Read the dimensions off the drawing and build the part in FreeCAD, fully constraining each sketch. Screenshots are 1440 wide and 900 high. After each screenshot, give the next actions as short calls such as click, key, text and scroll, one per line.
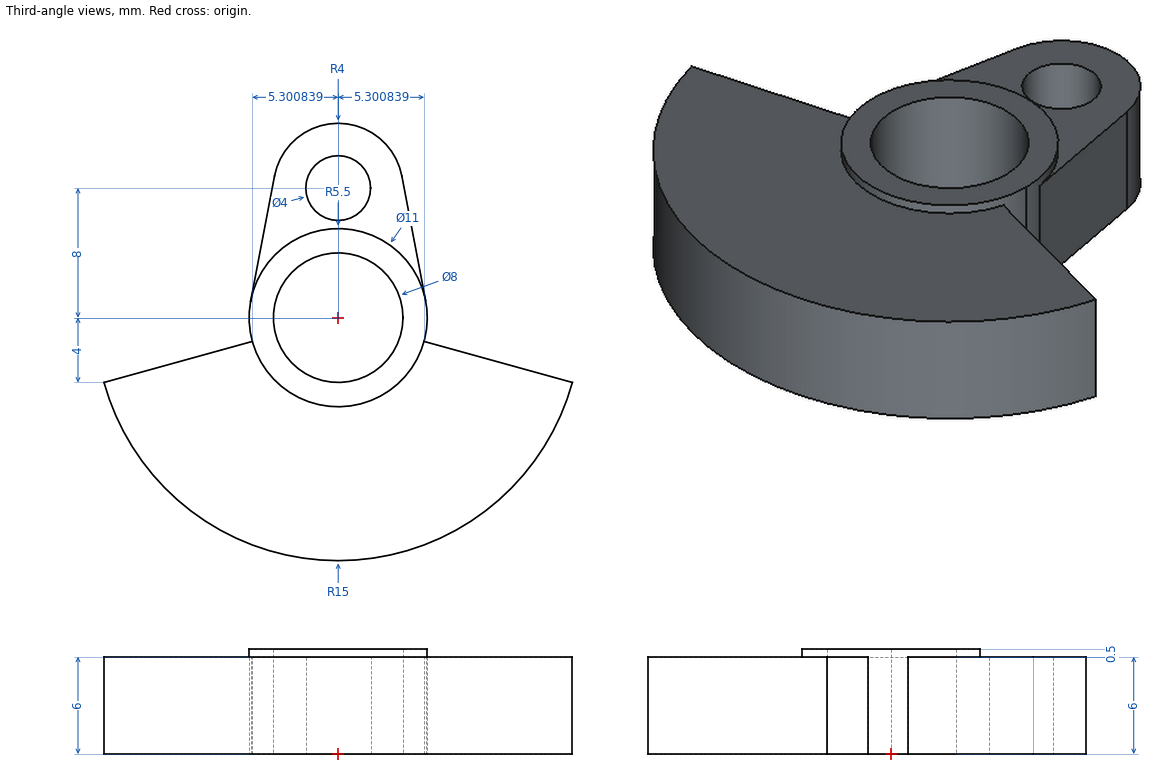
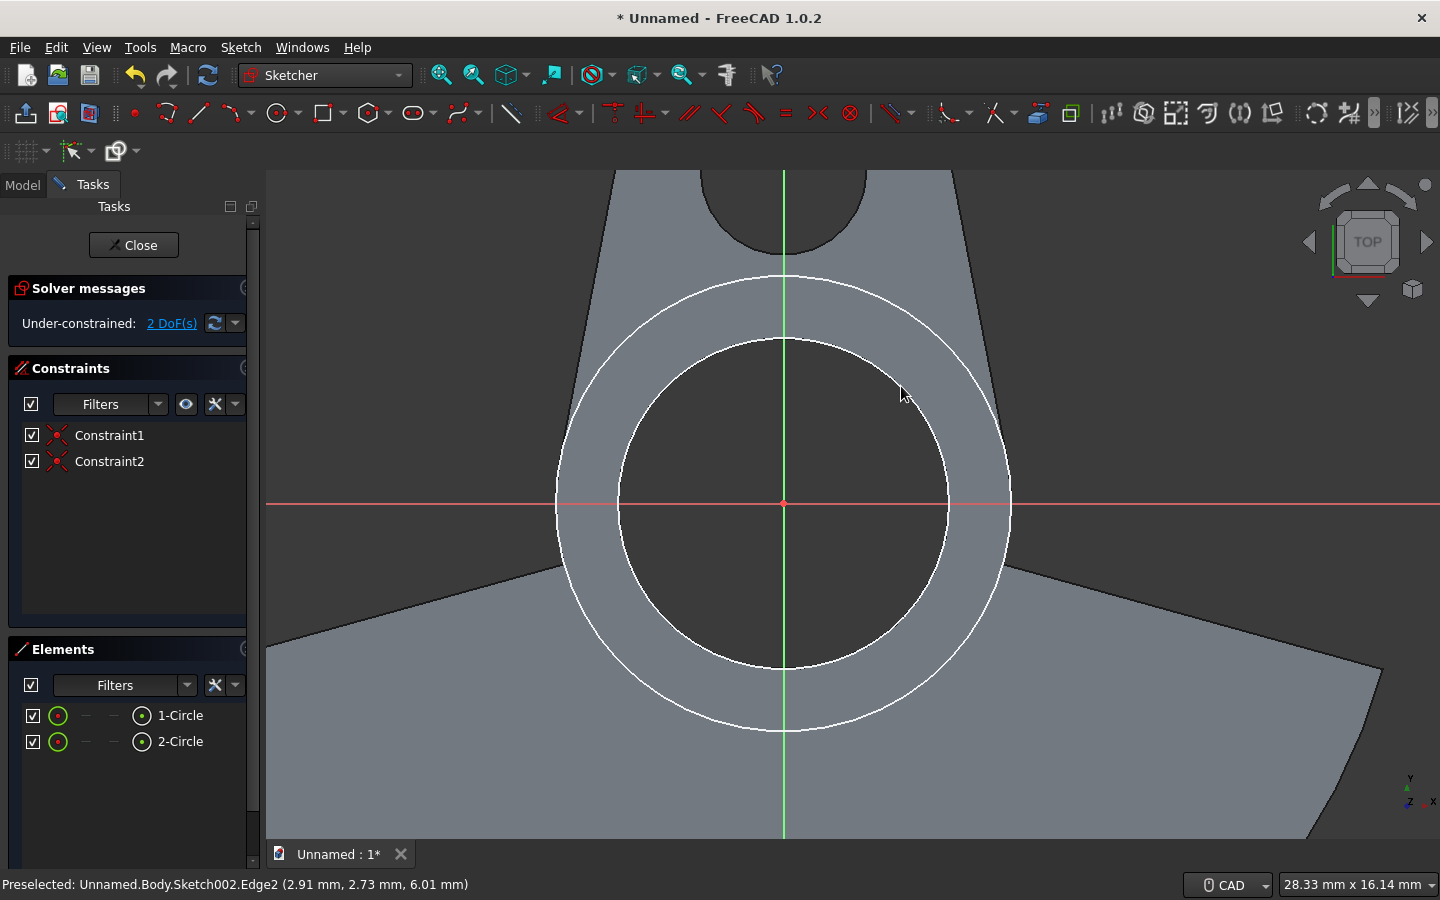
click(558, 114)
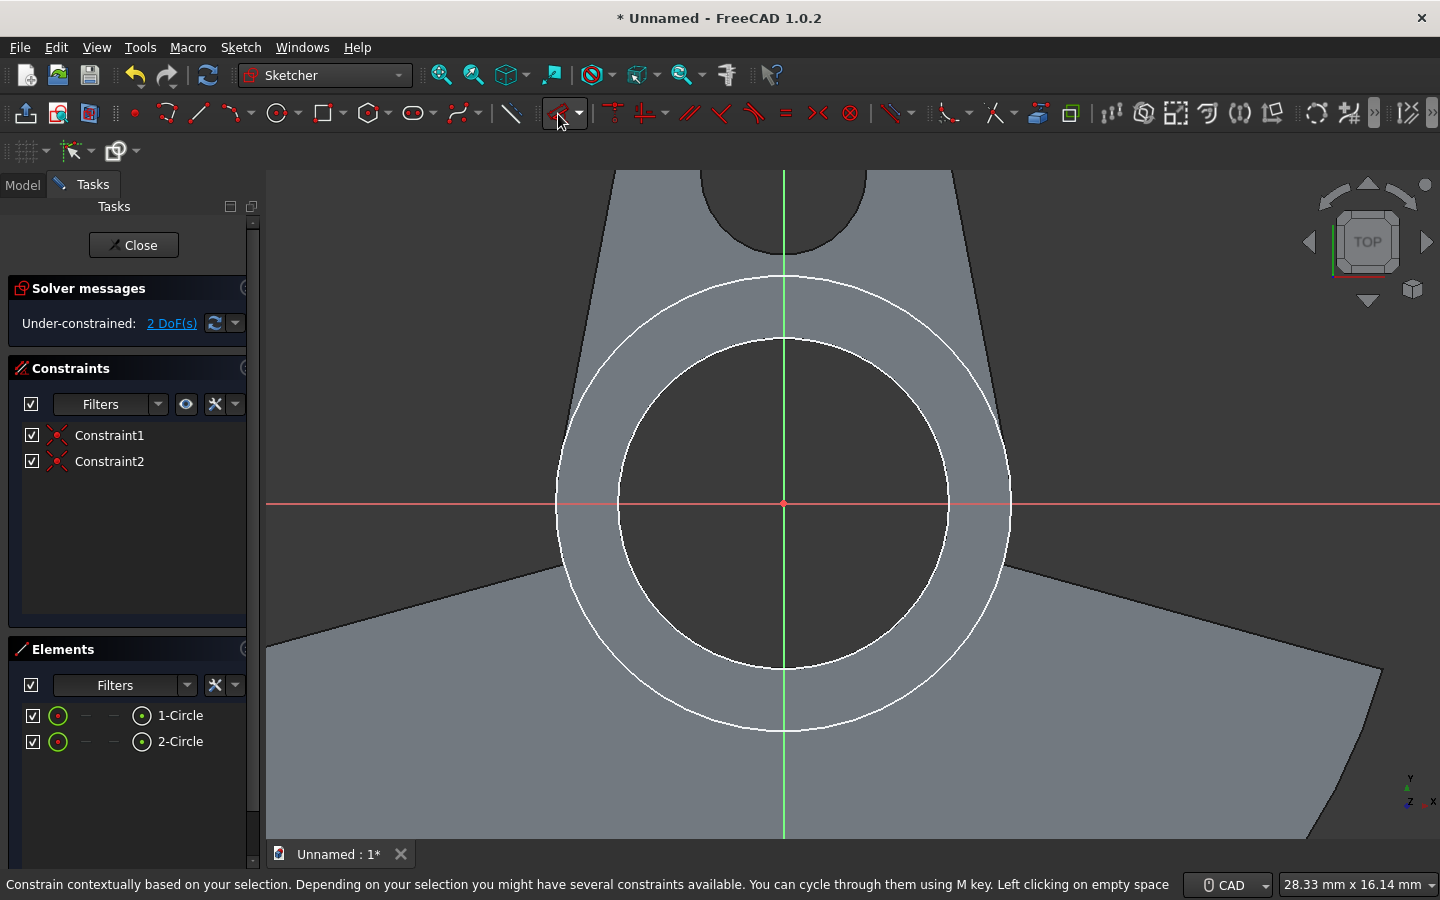
click(944, 342)
click(967, 319)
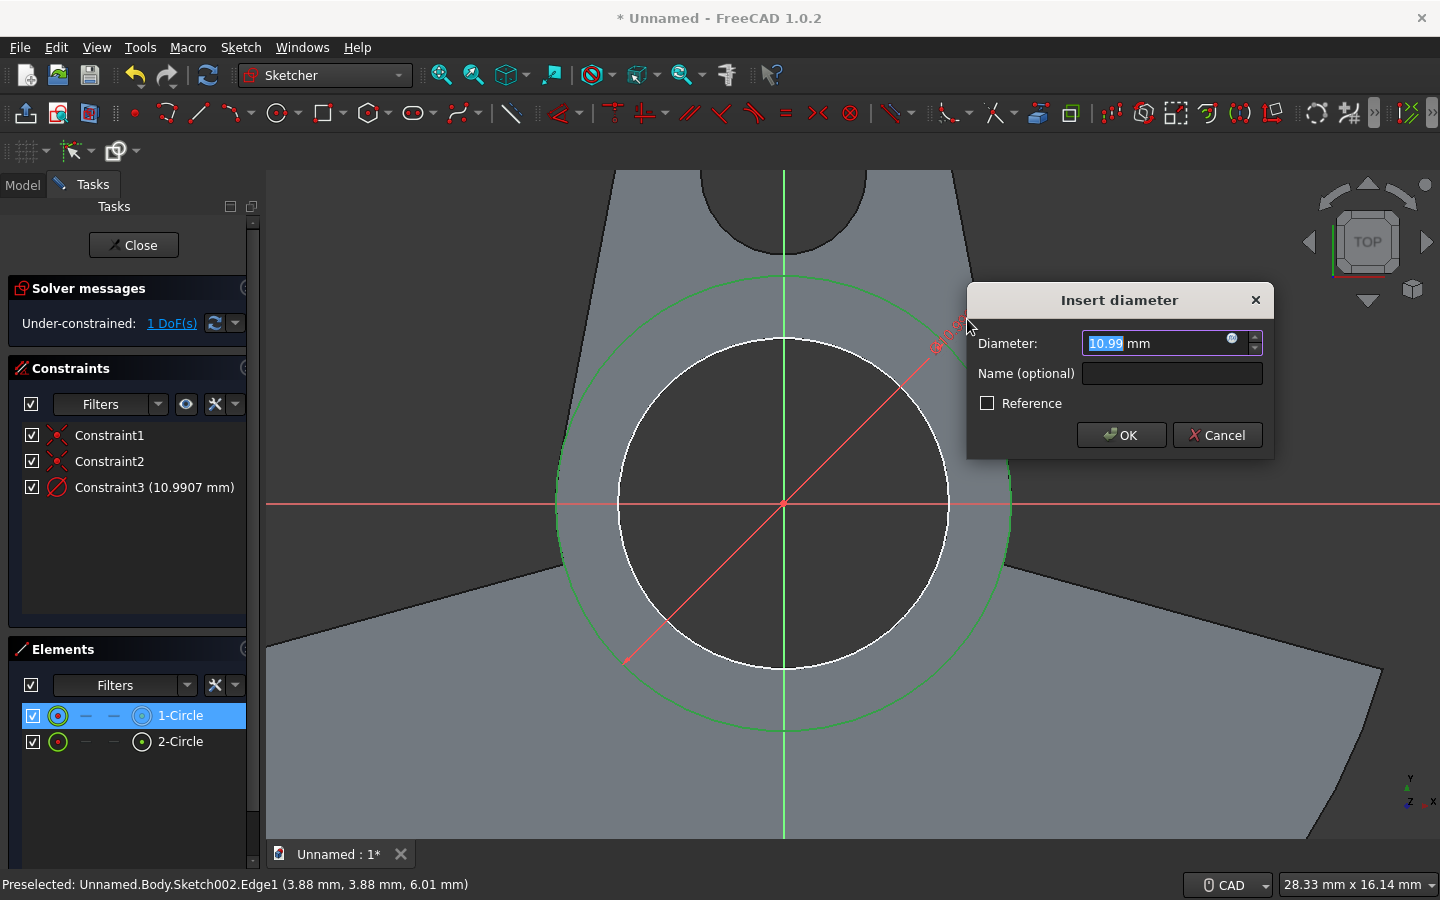
text(11)
key(Return)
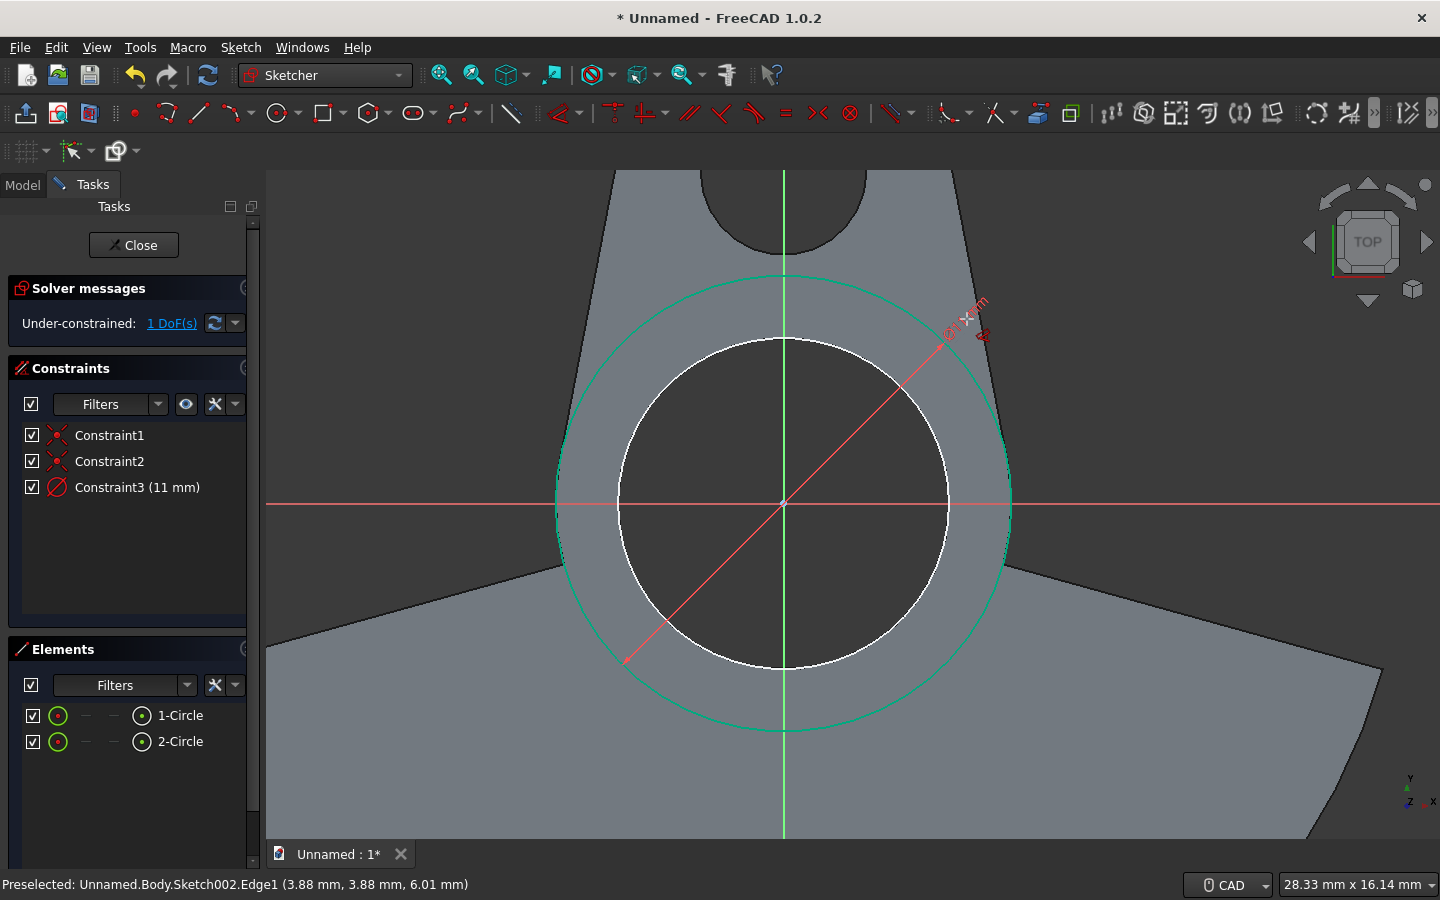
click(900, 386)
click(923, 363)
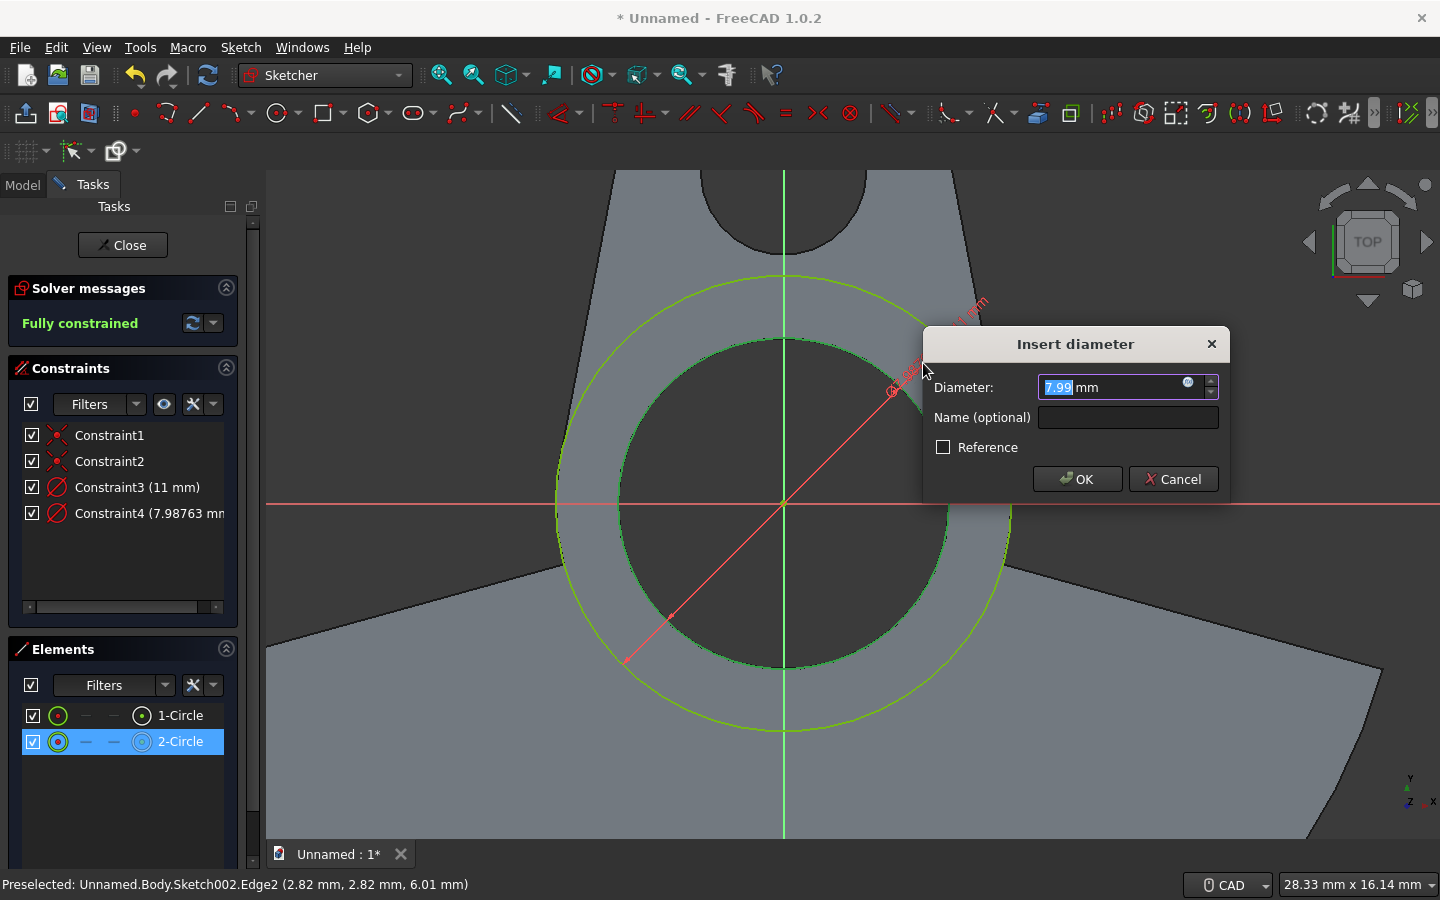
text(8)
key(Return)
key(Escape)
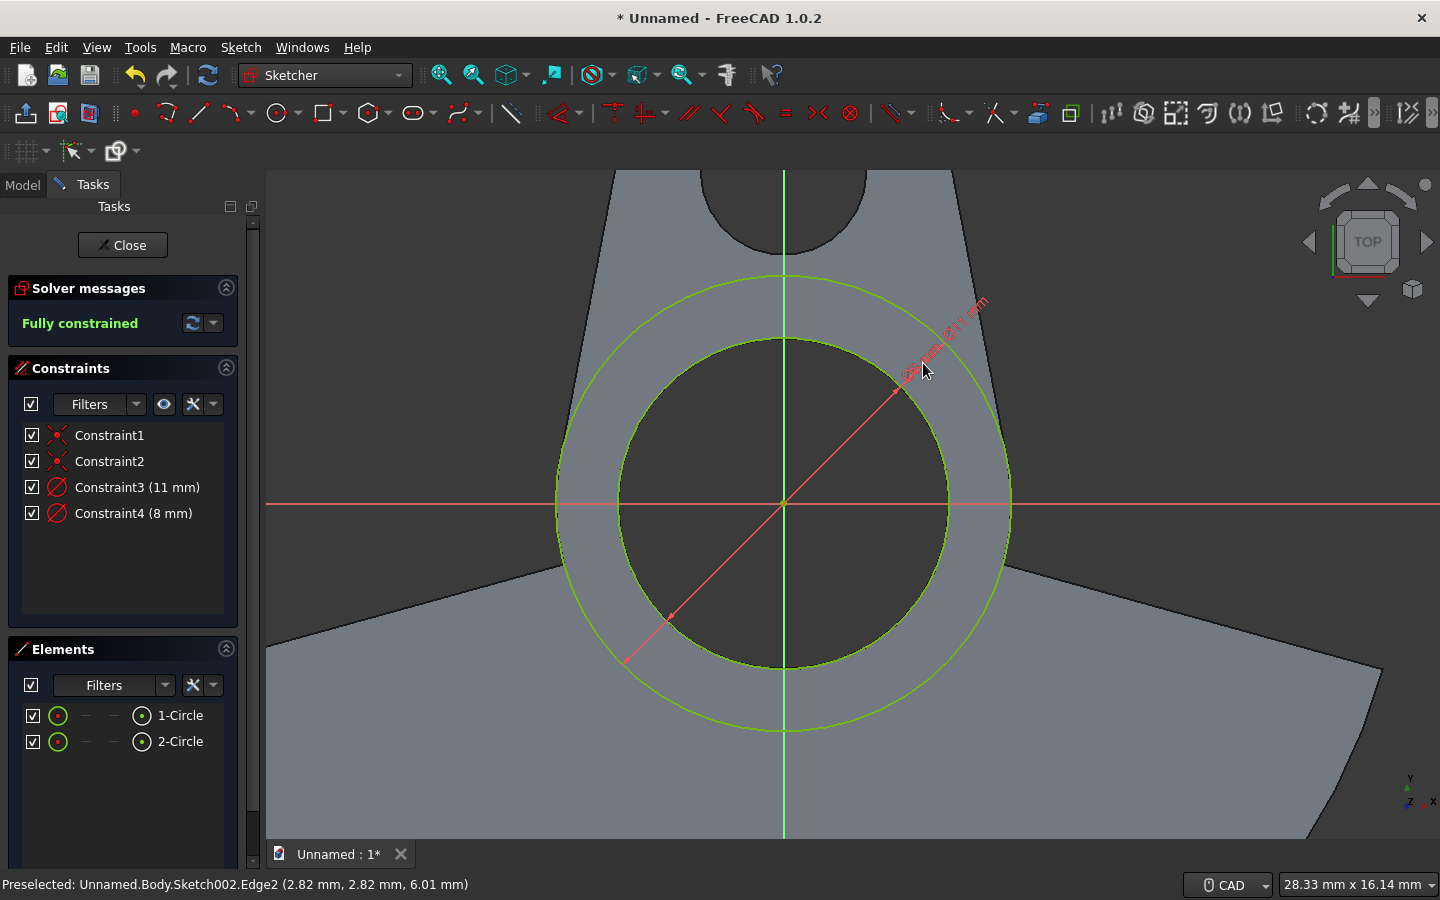
click(123, 245)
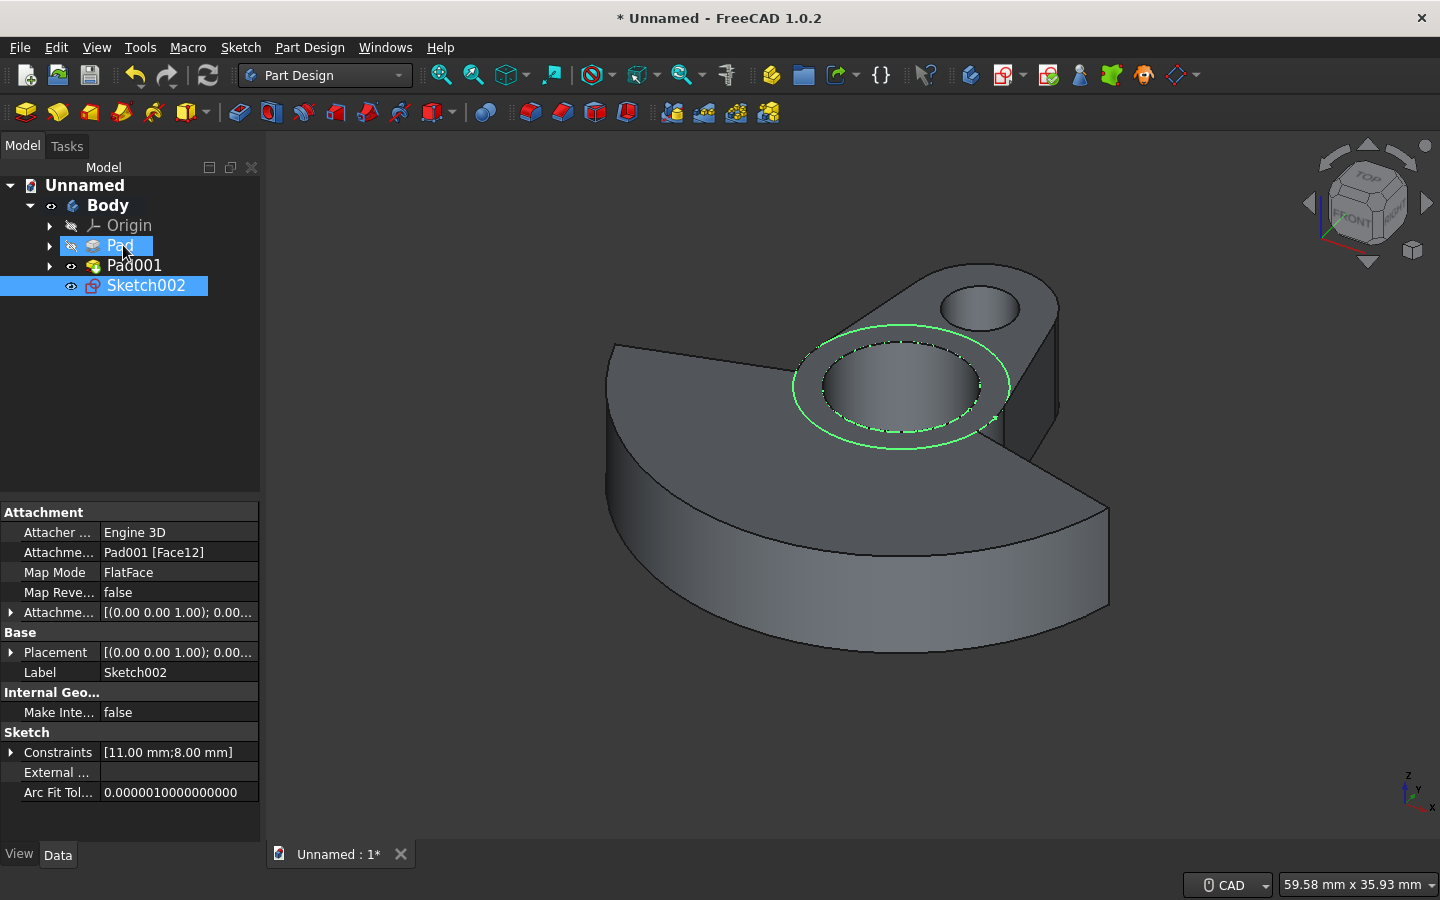
click(26, 112)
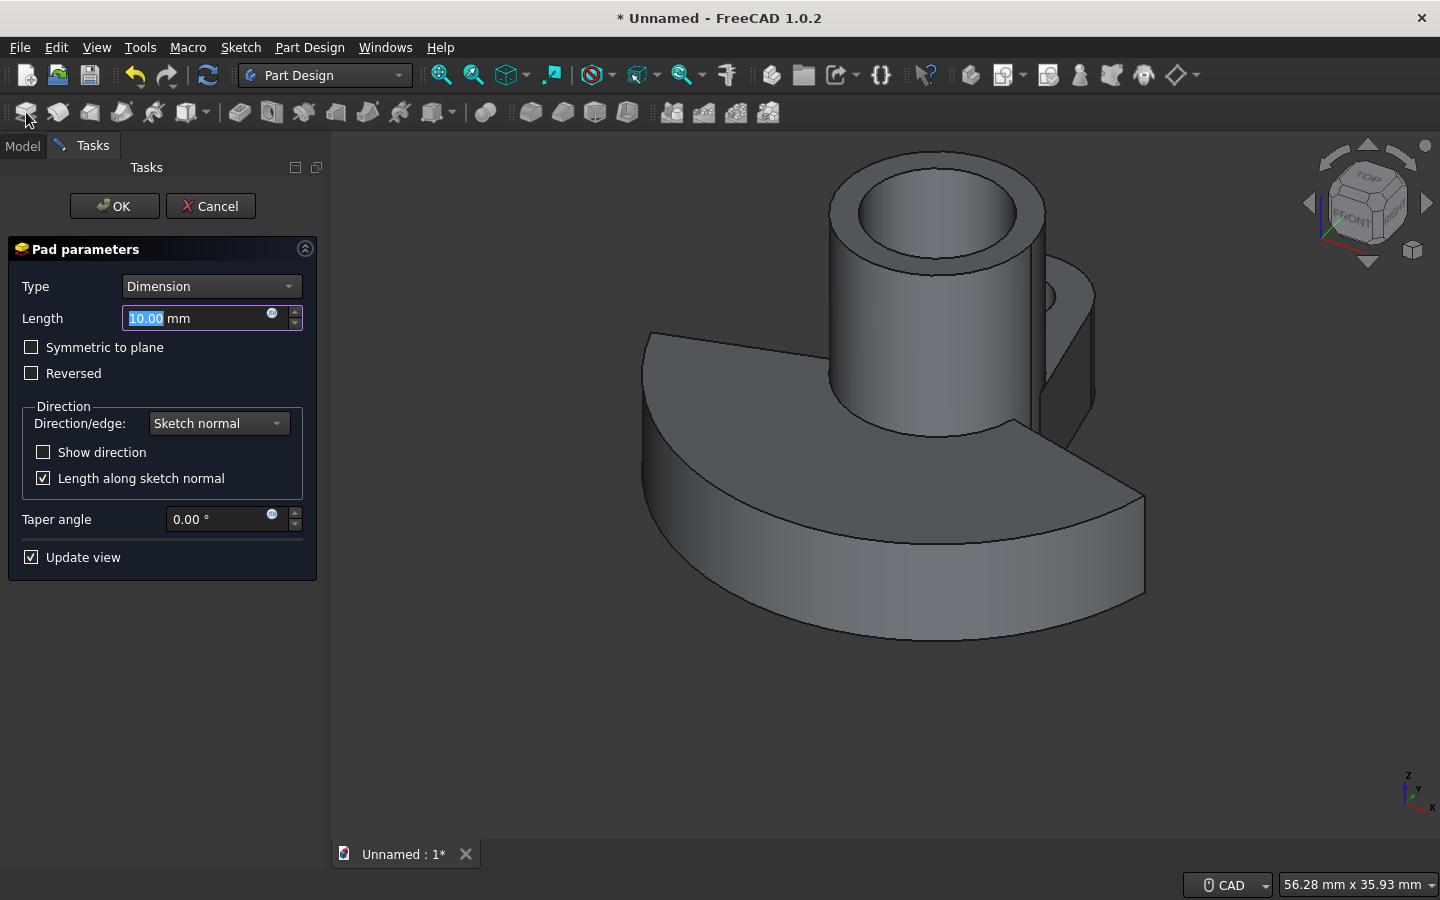
text(0.5)
key(Tab)